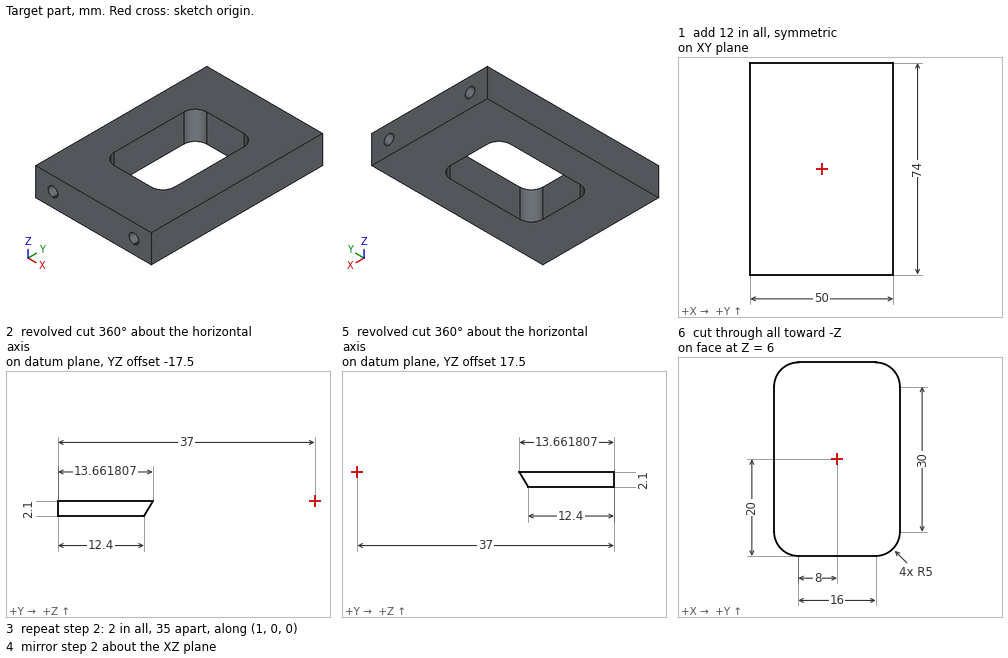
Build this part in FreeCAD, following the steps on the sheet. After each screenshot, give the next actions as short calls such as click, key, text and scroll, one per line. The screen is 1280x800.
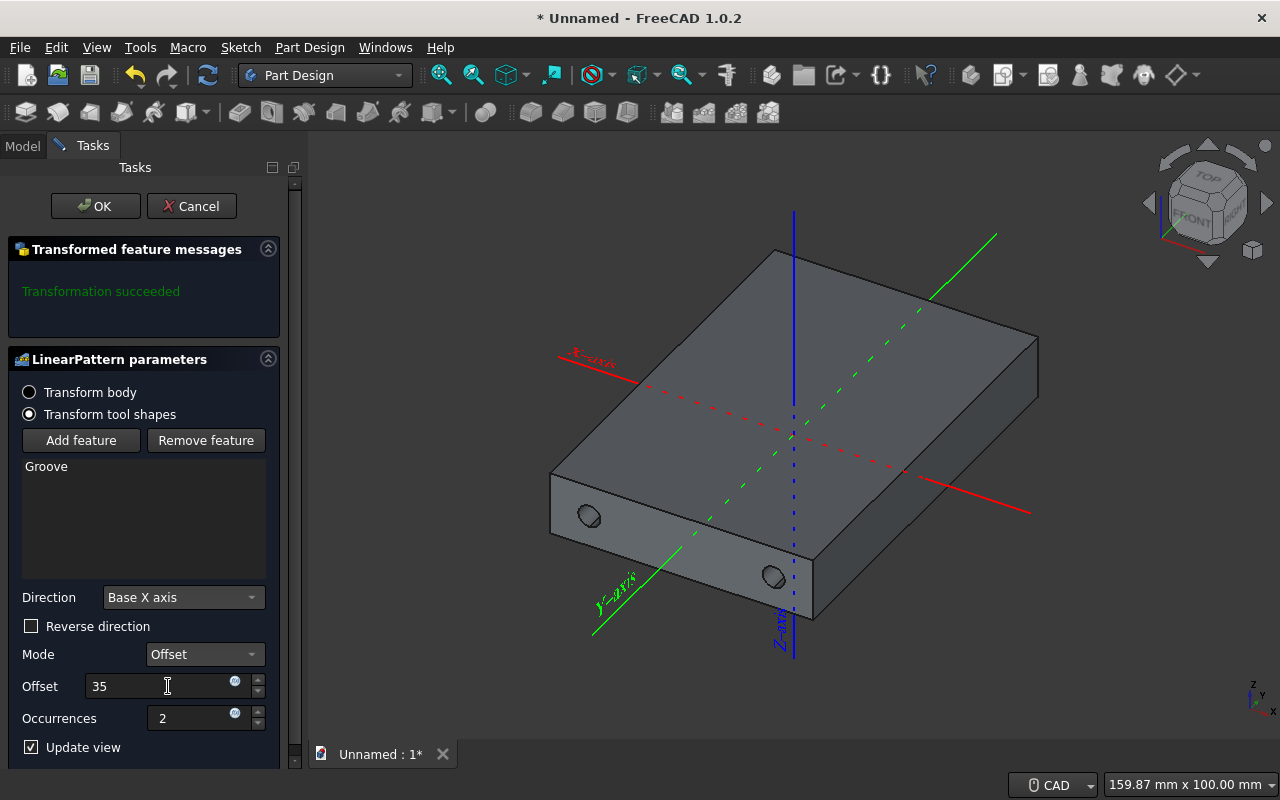
triple_click(198, 718)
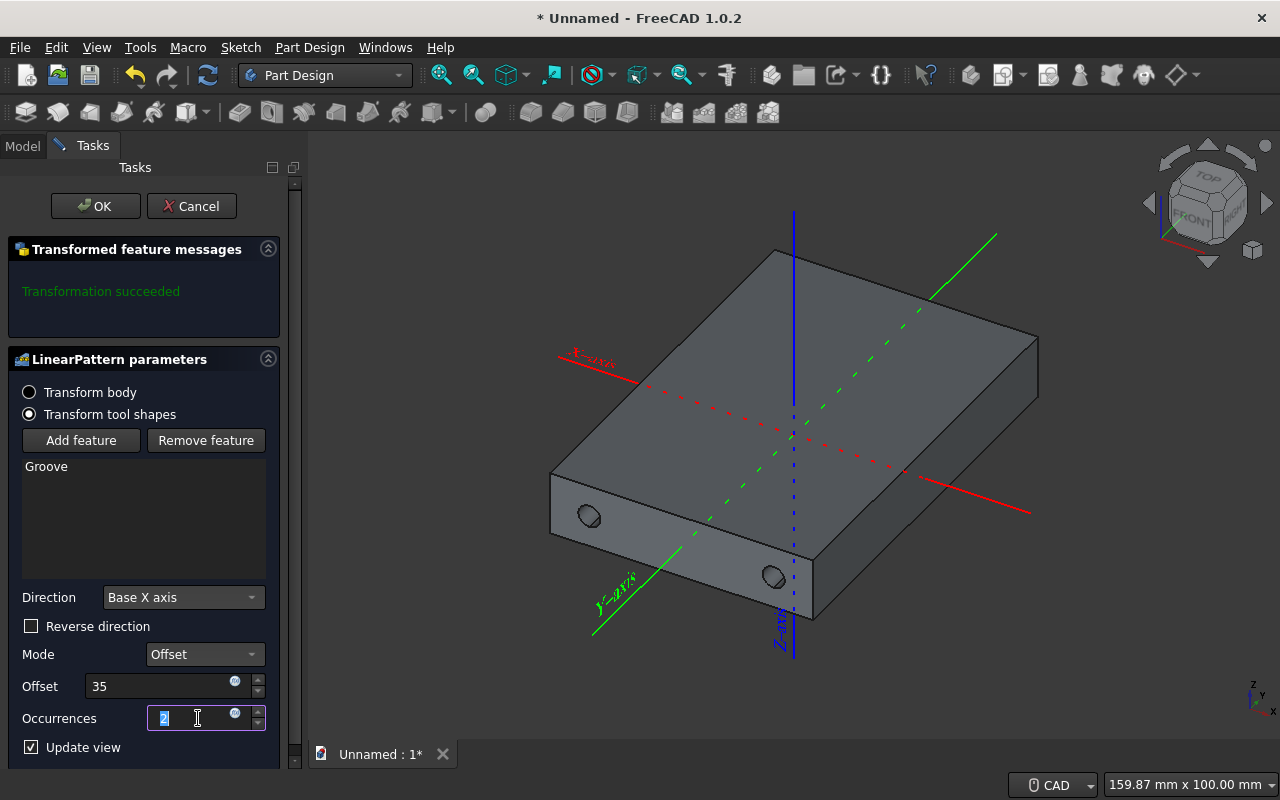
text(2)
key(Tab)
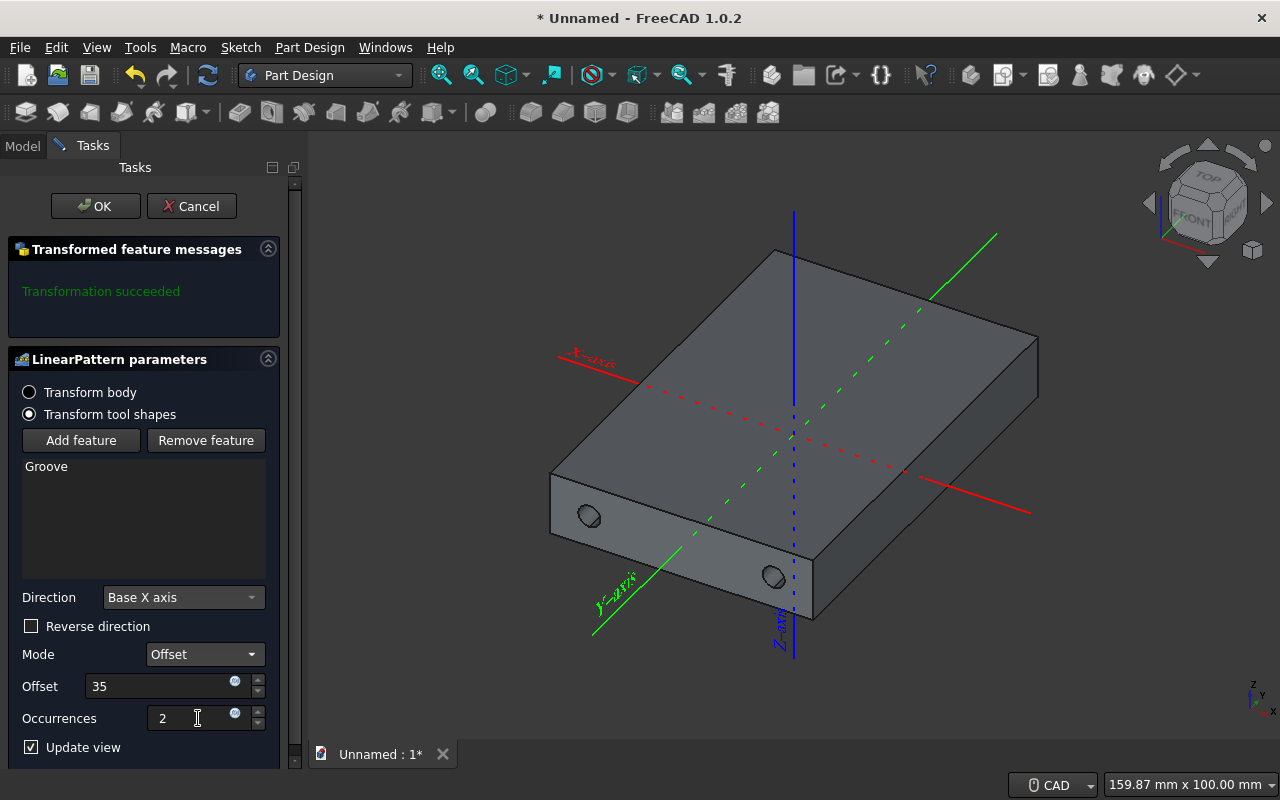
click(96, 206)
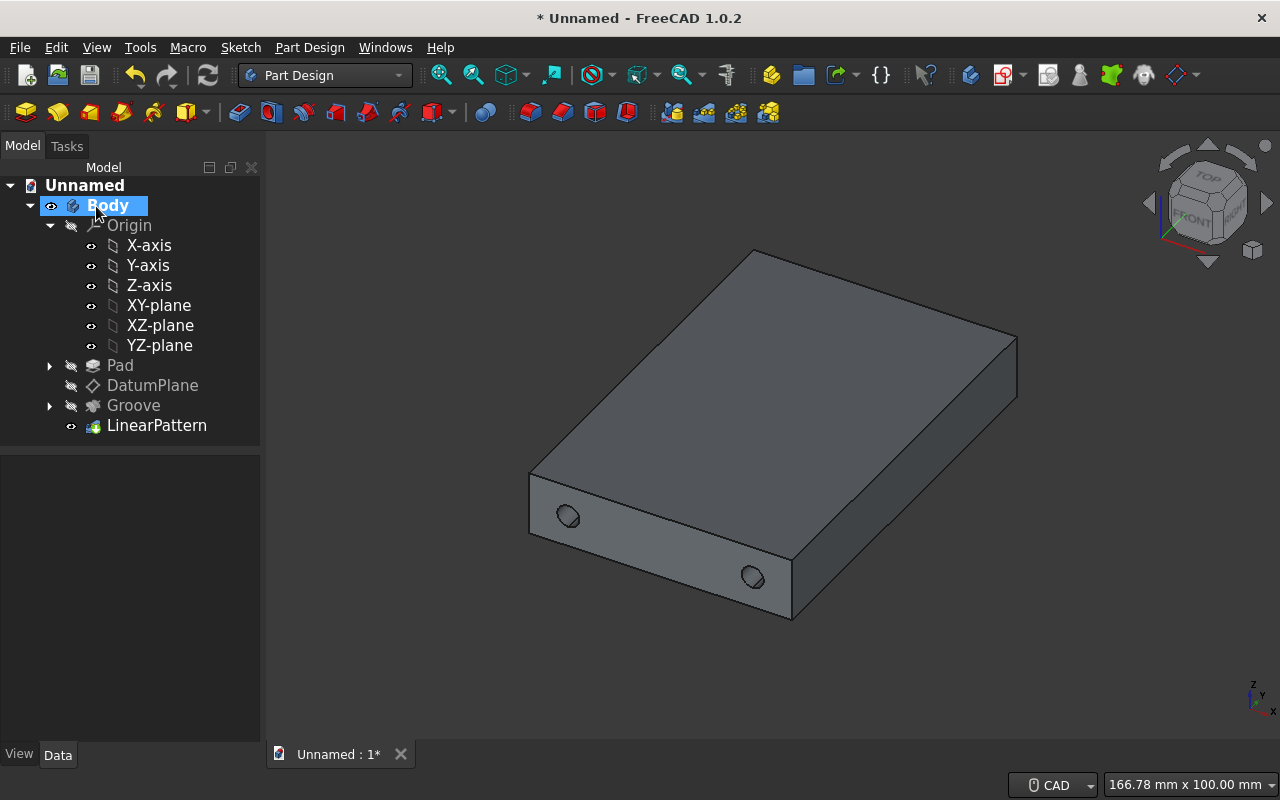
click(116, 406)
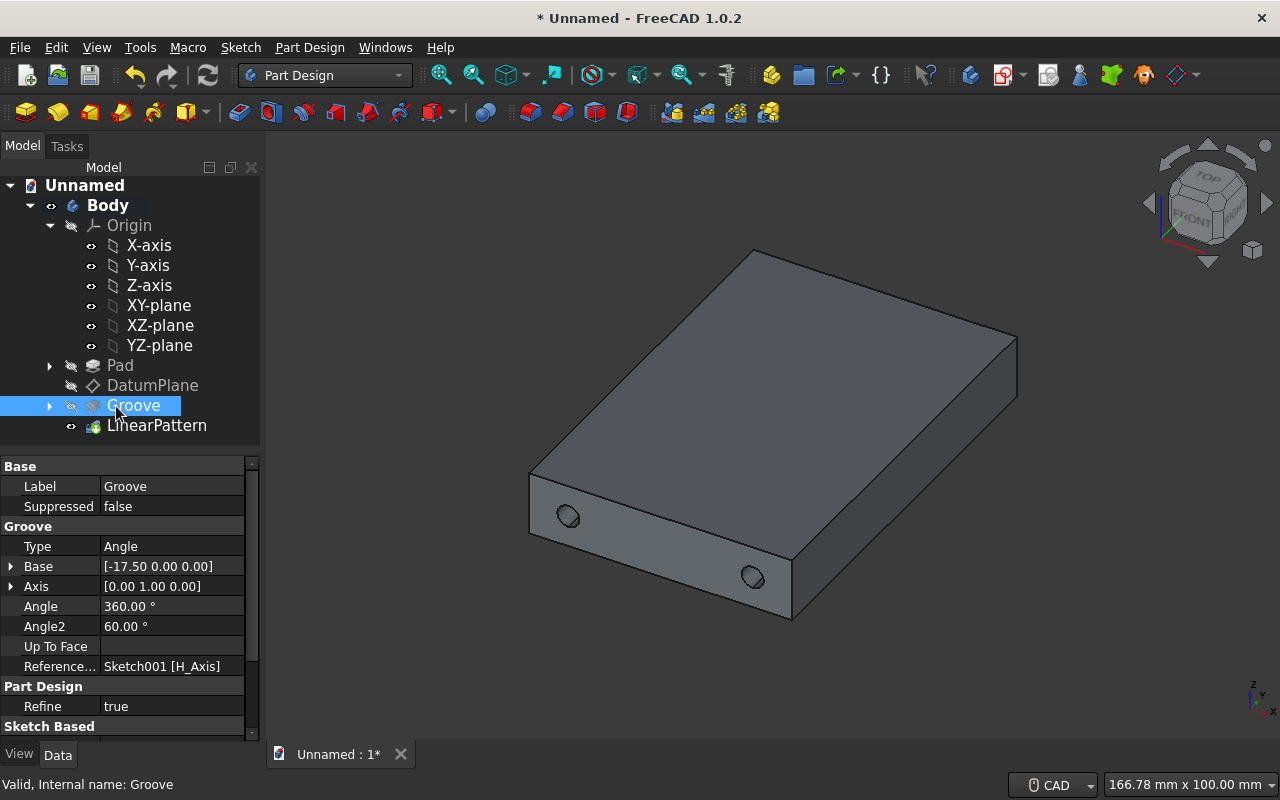
click(672, 112)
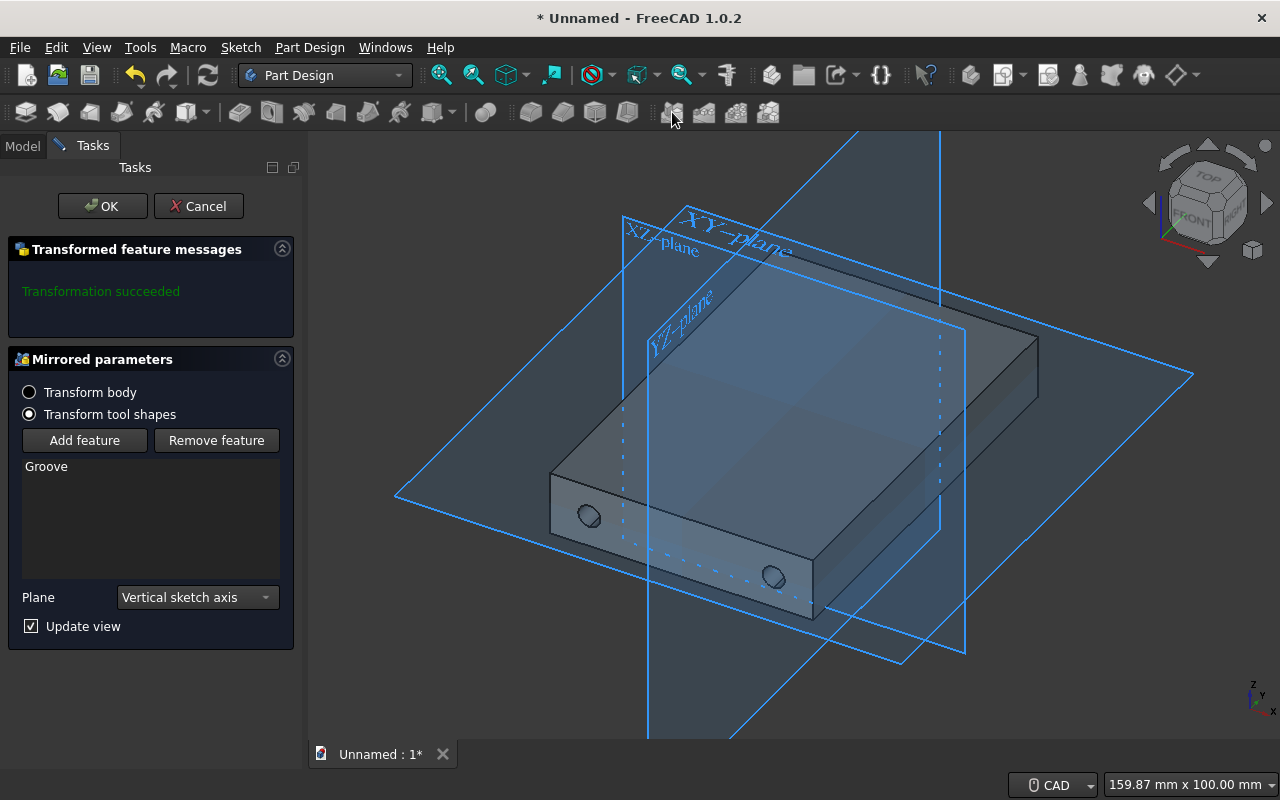
click(198, 598)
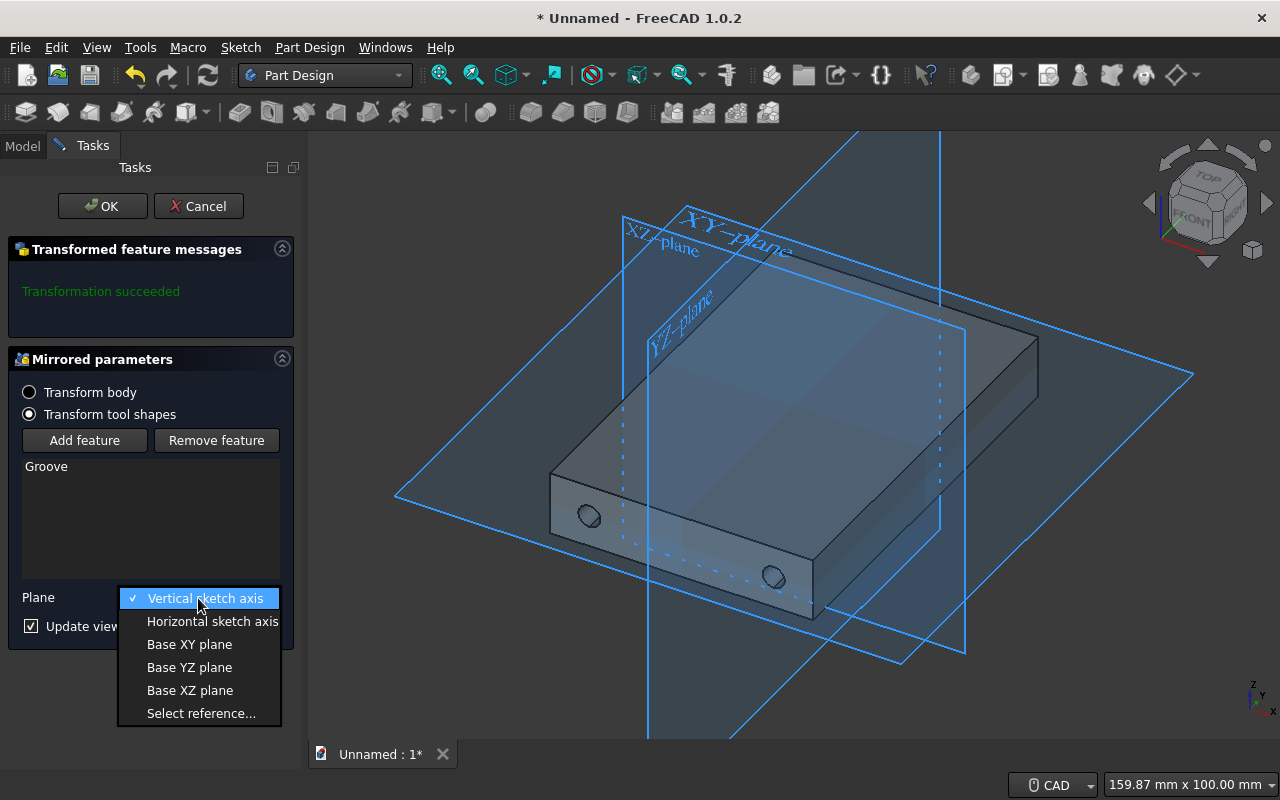
click(198, 690)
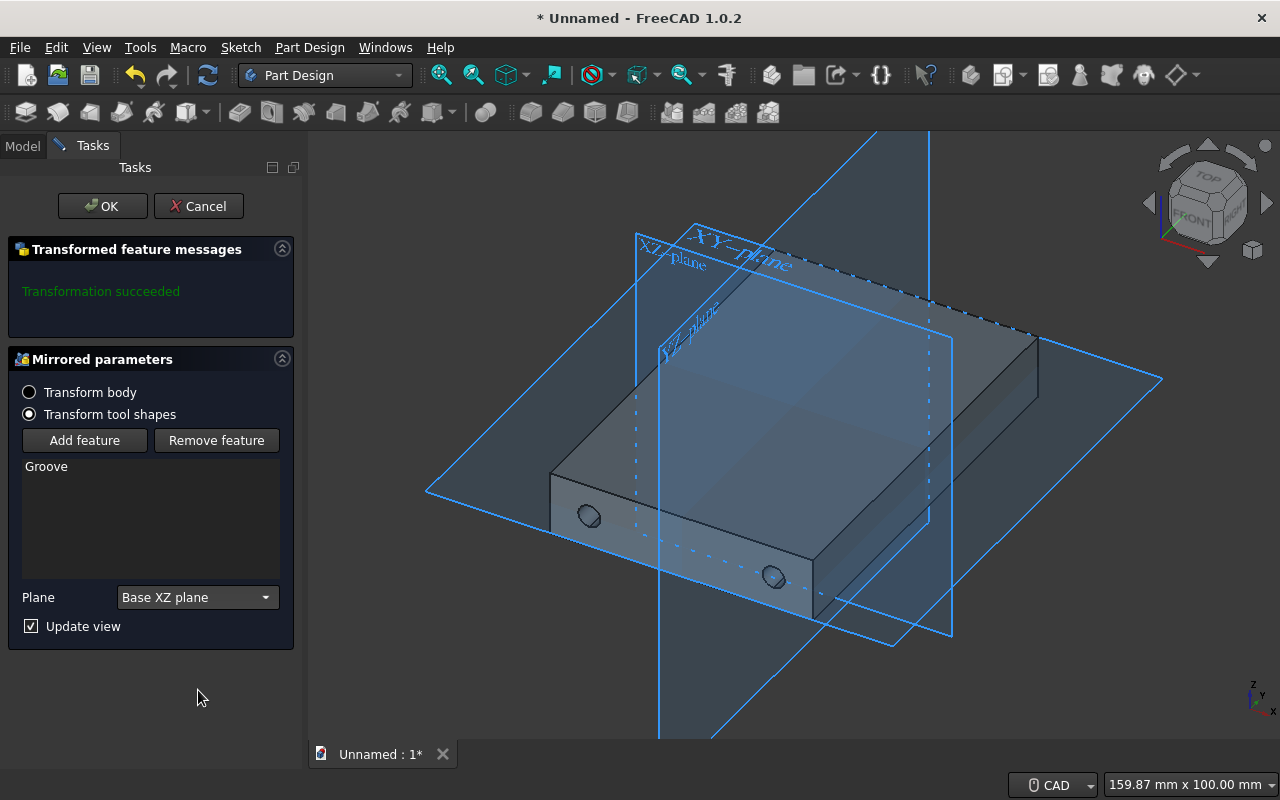
click(103, 206)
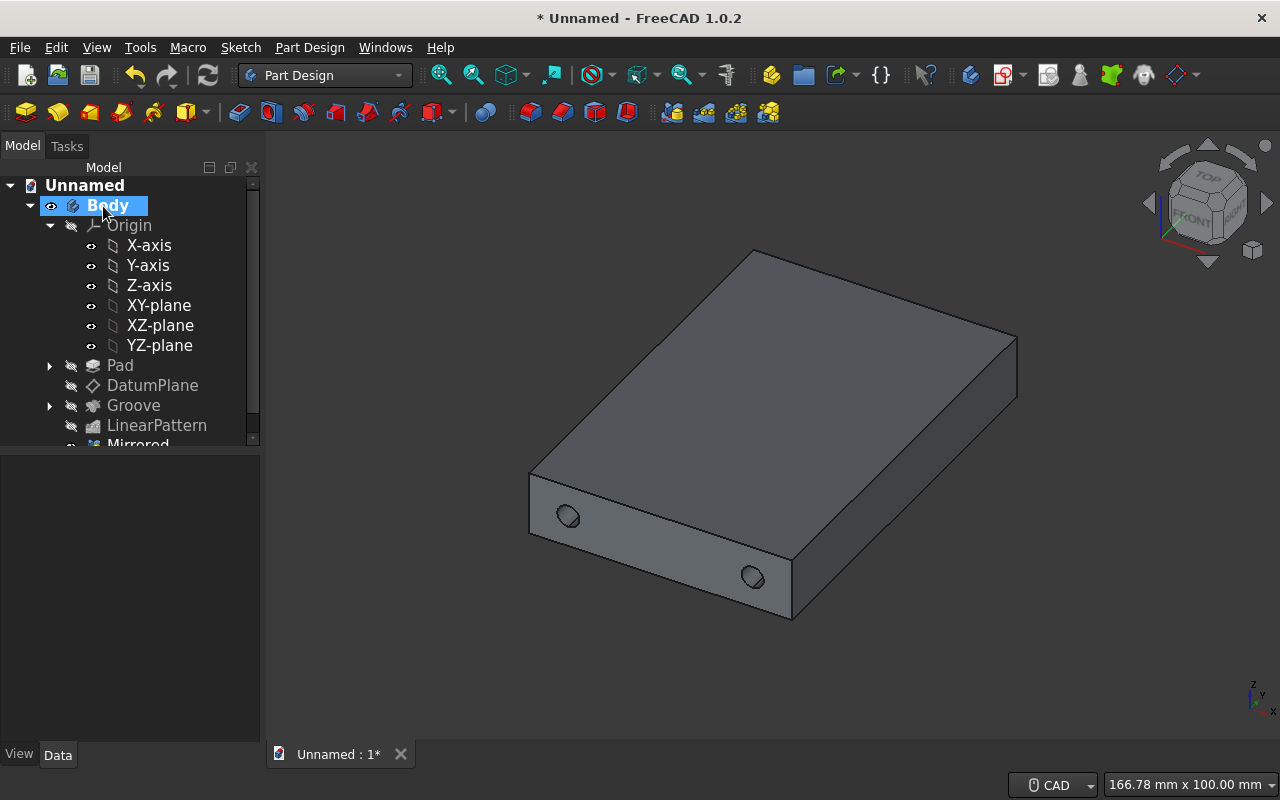
click(136, 346)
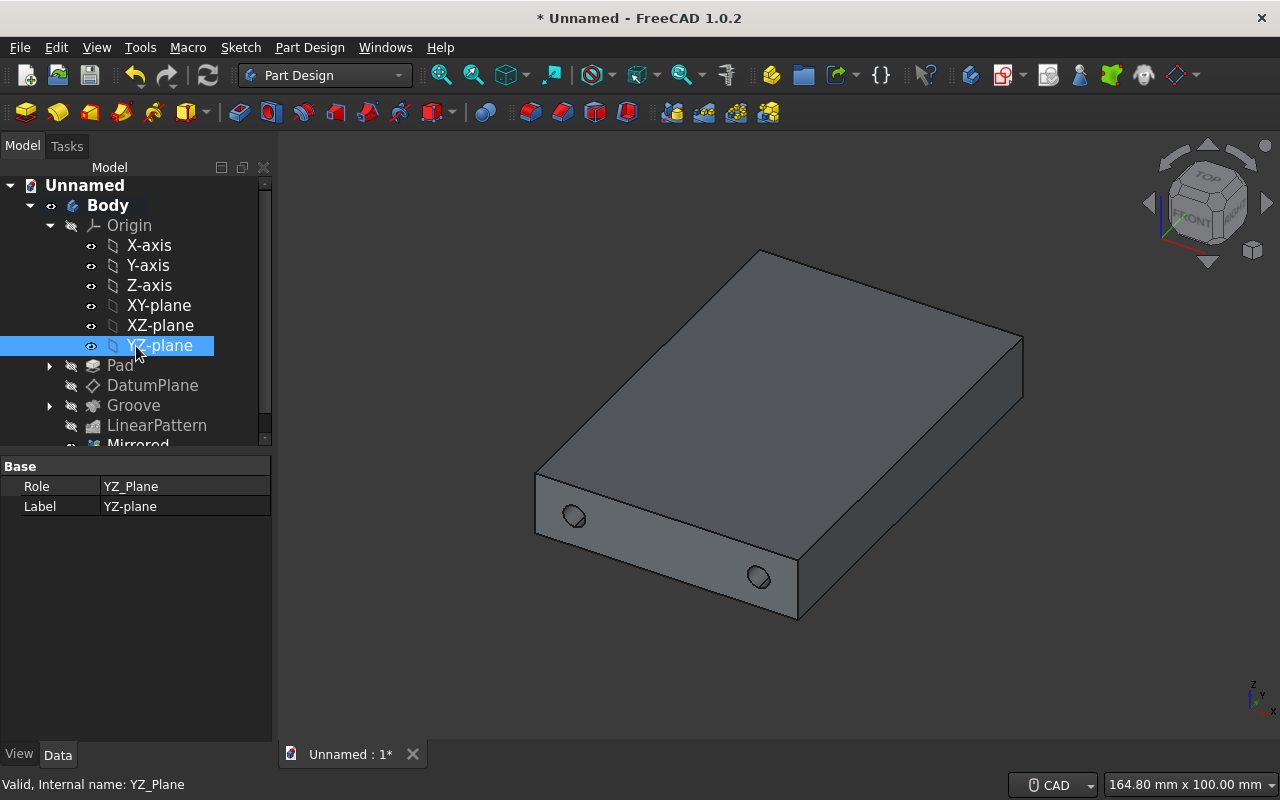
click(1176, 76)